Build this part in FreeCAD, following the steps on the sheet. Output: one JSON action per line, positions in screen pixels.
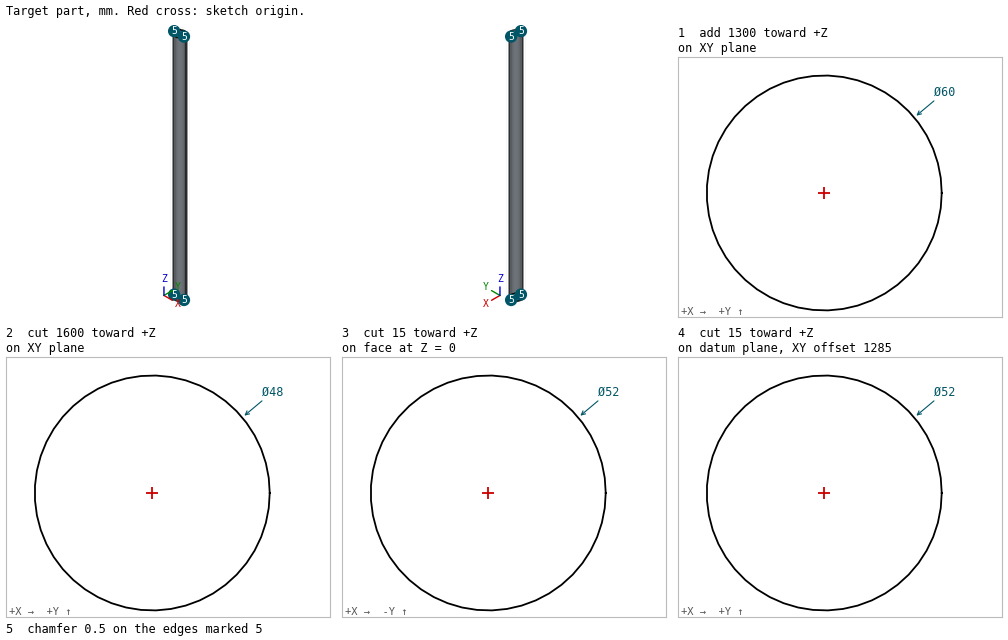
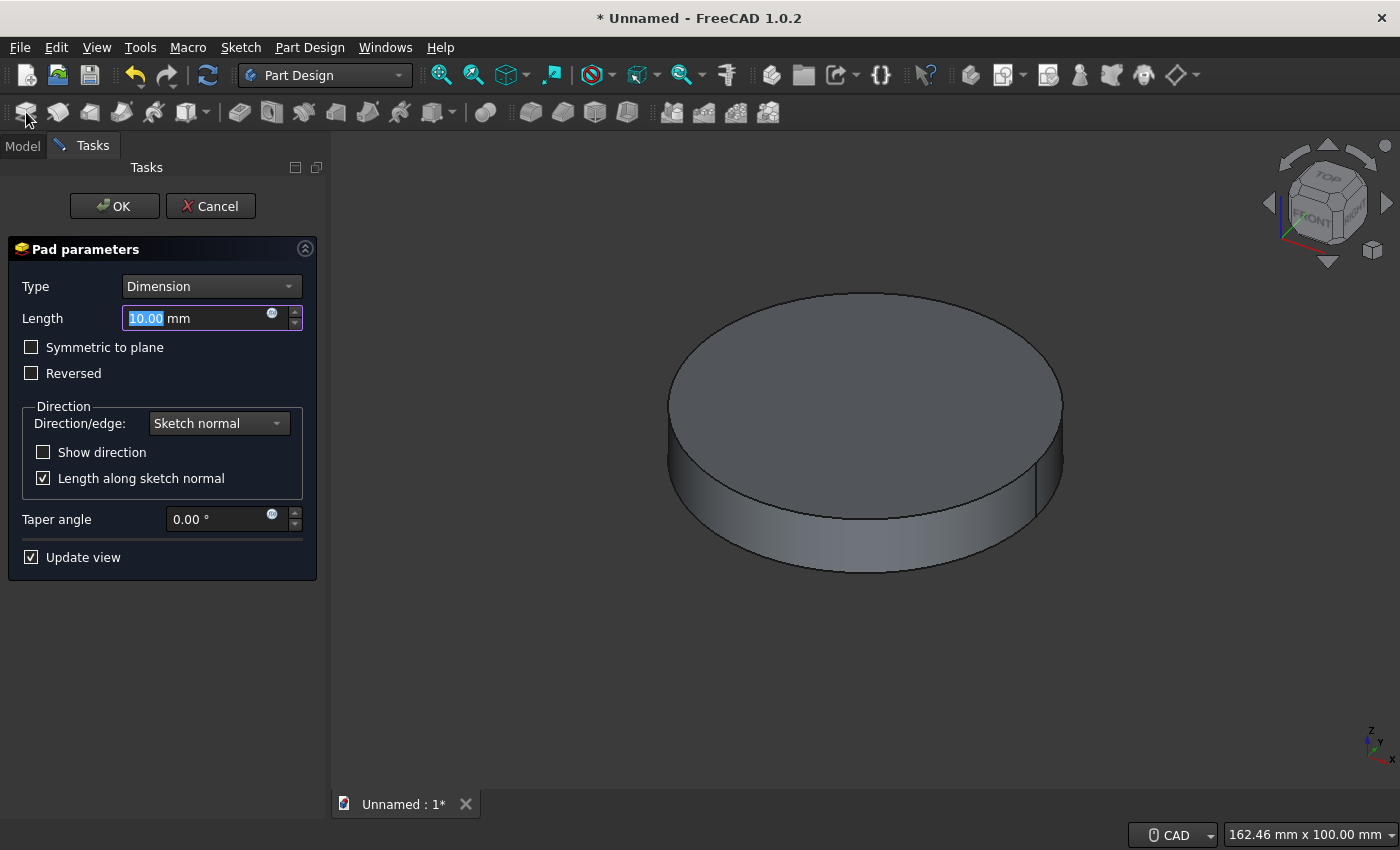
{"action": "type", "text": "1300"}
{"action": "key", "text": "Tab"}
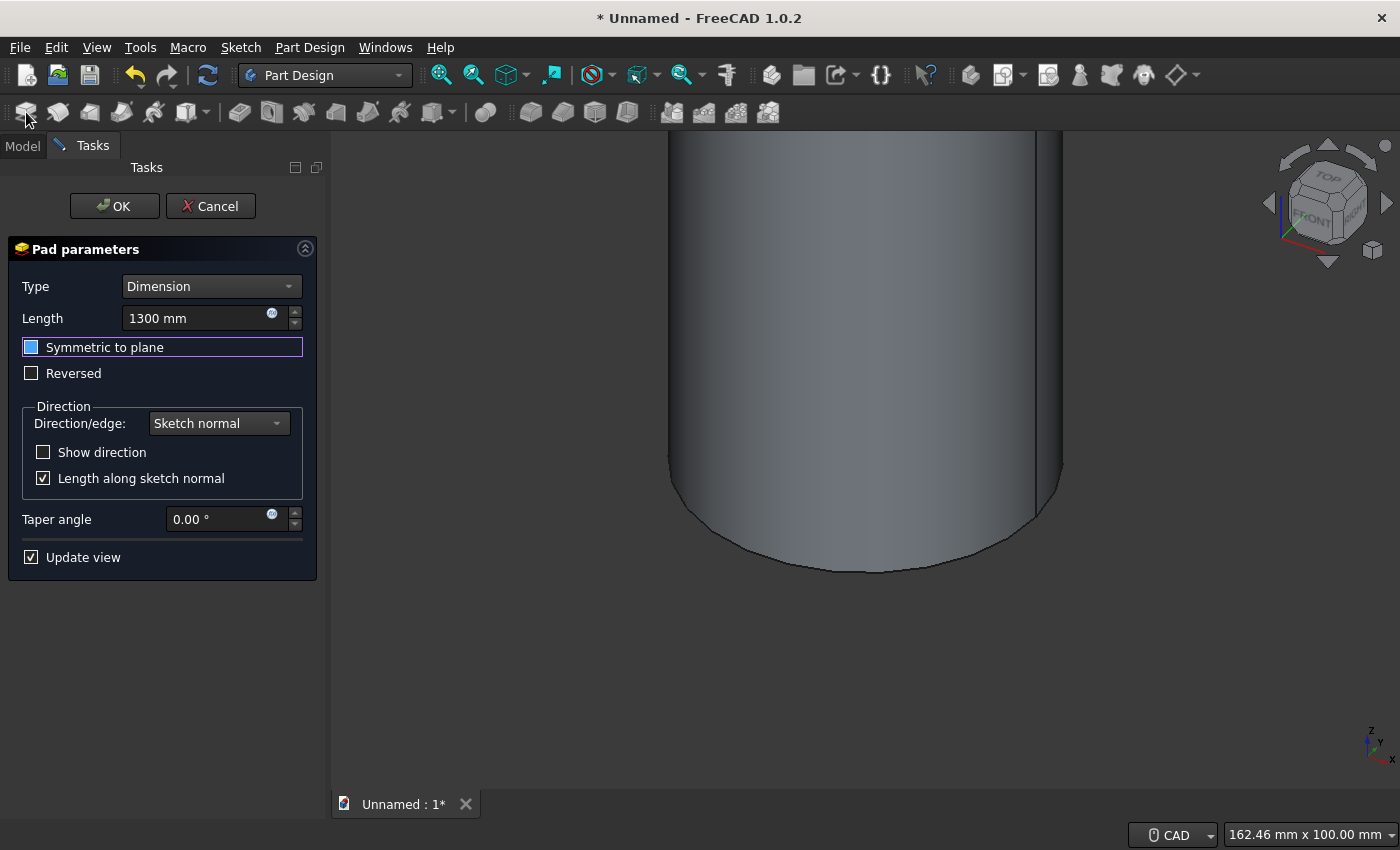
{"action": "left_click", "coordinate": [115, 206]}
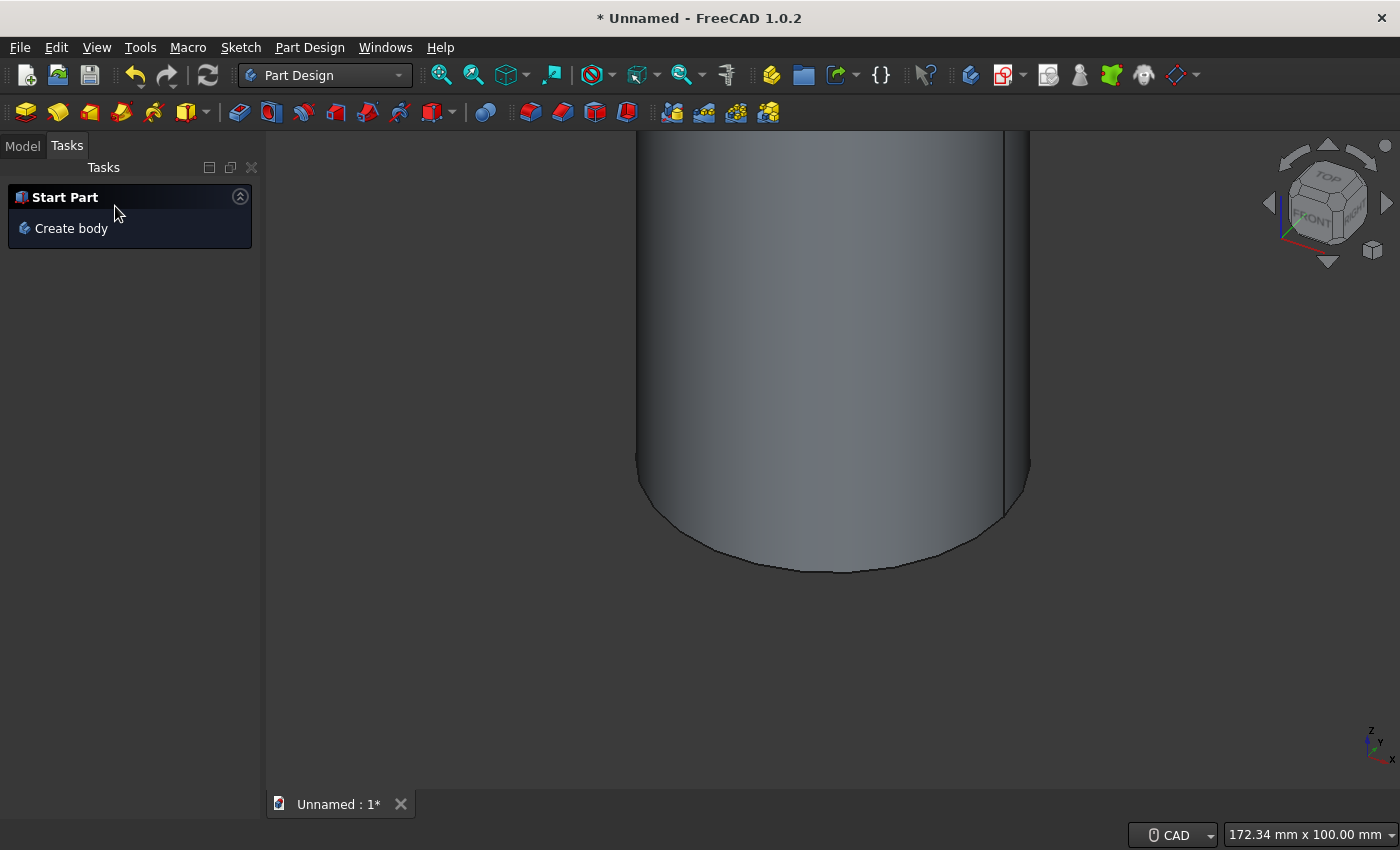
{"action": "left_click", "coordinate": [442, 76]}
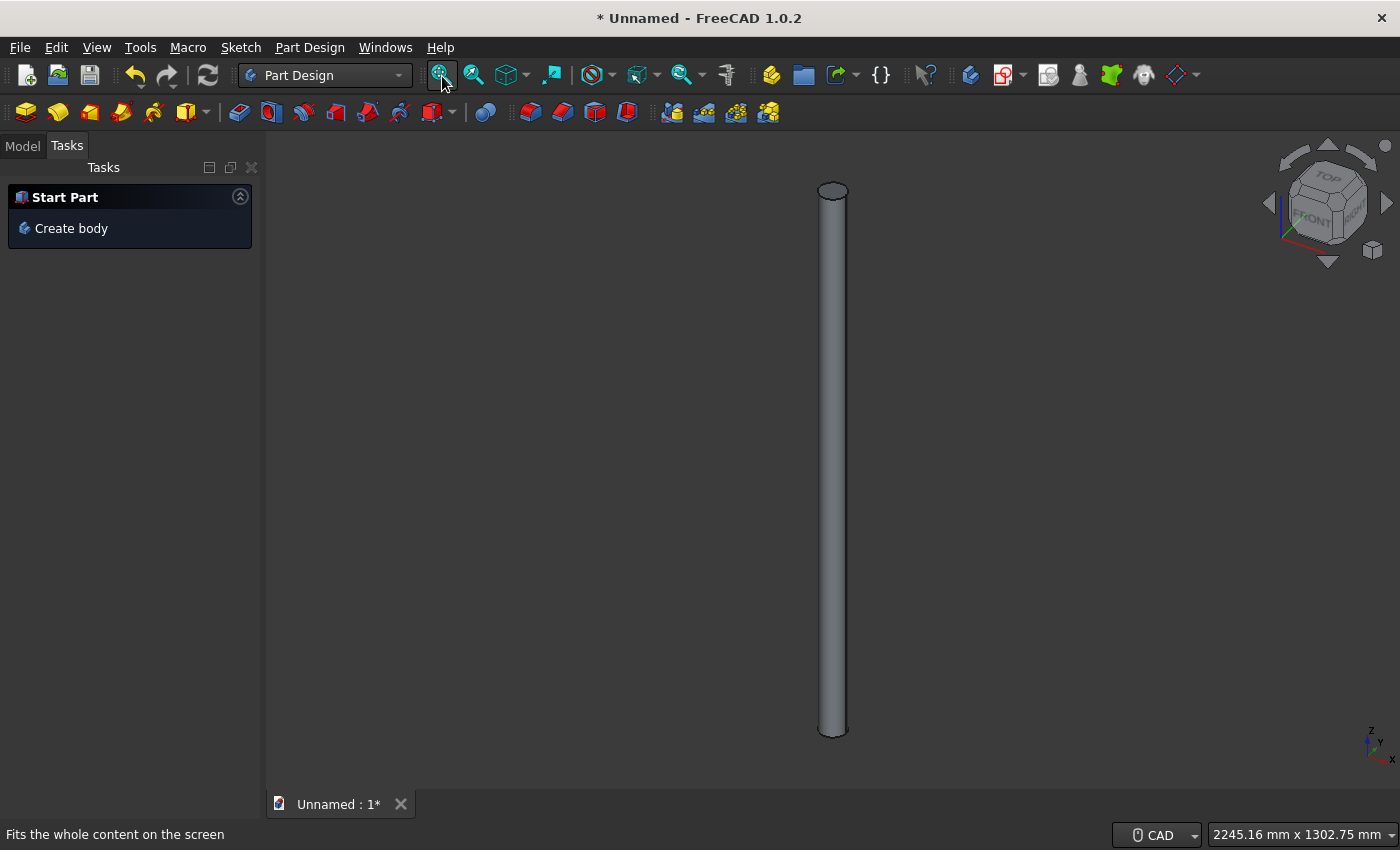
{"action": "left_click", "coordinate": [1004, 76]}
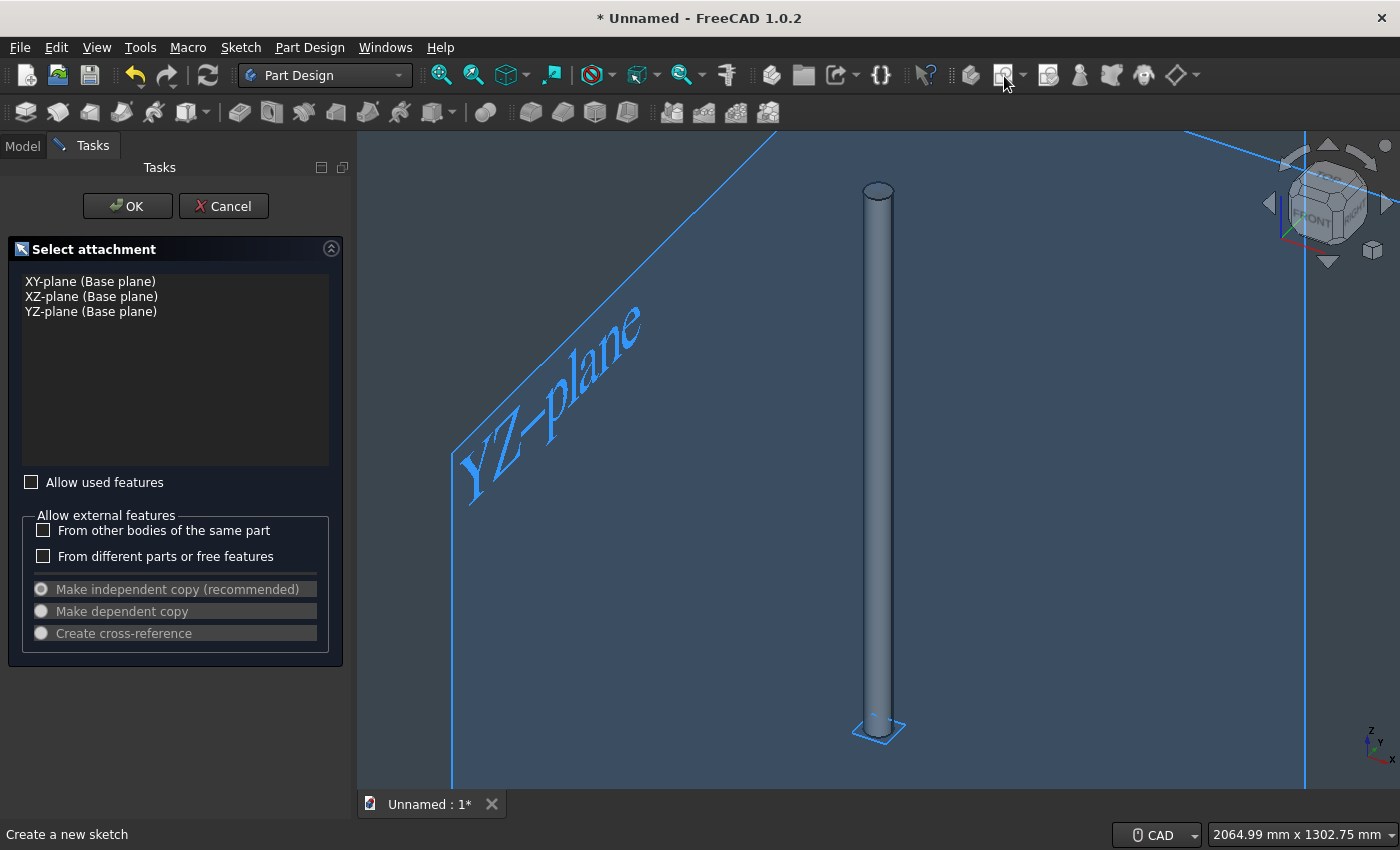
{"action": "left_click", "coordinate": [82, 282]}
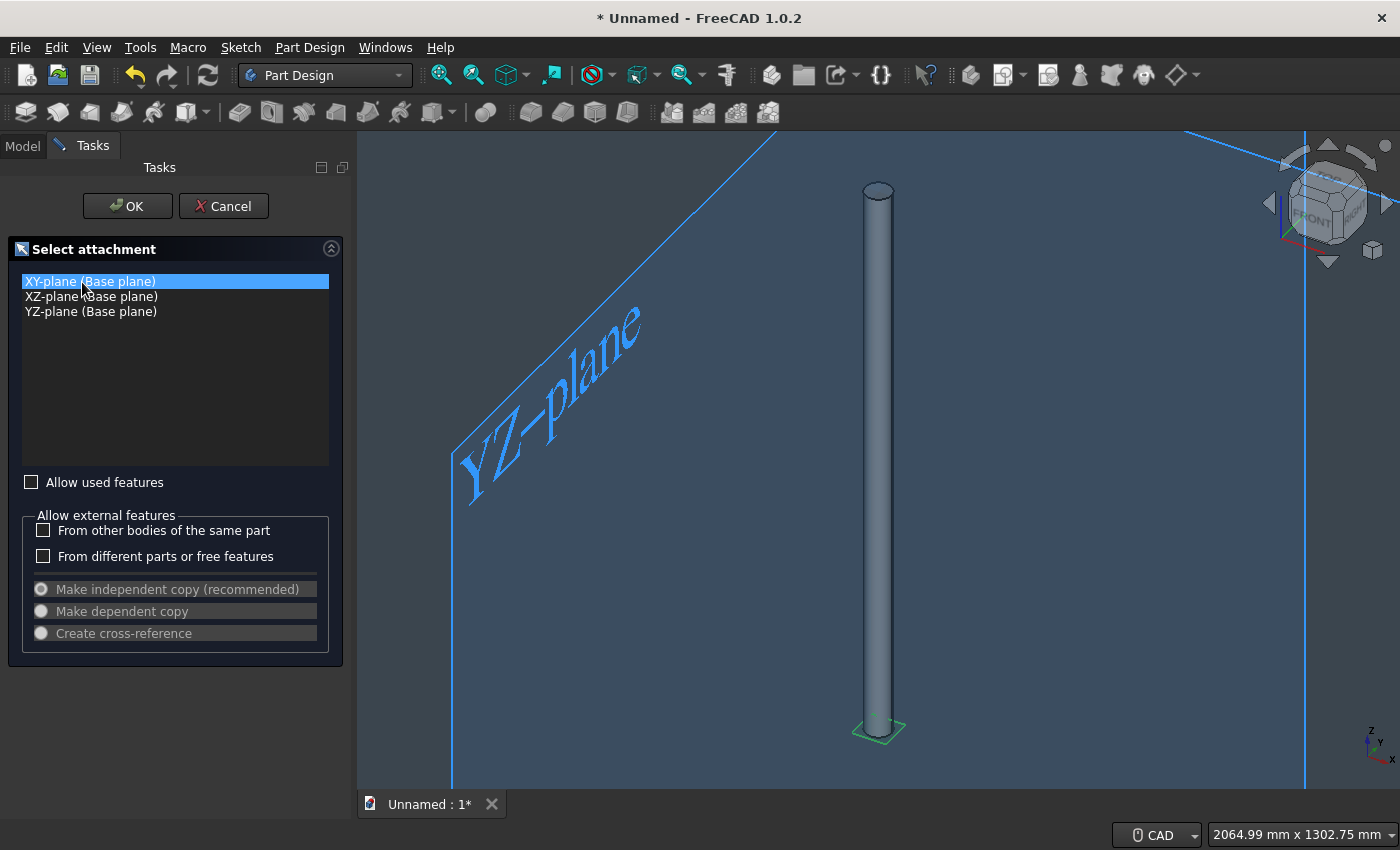
{"action": "left_click", "coordinate": [128, 206]}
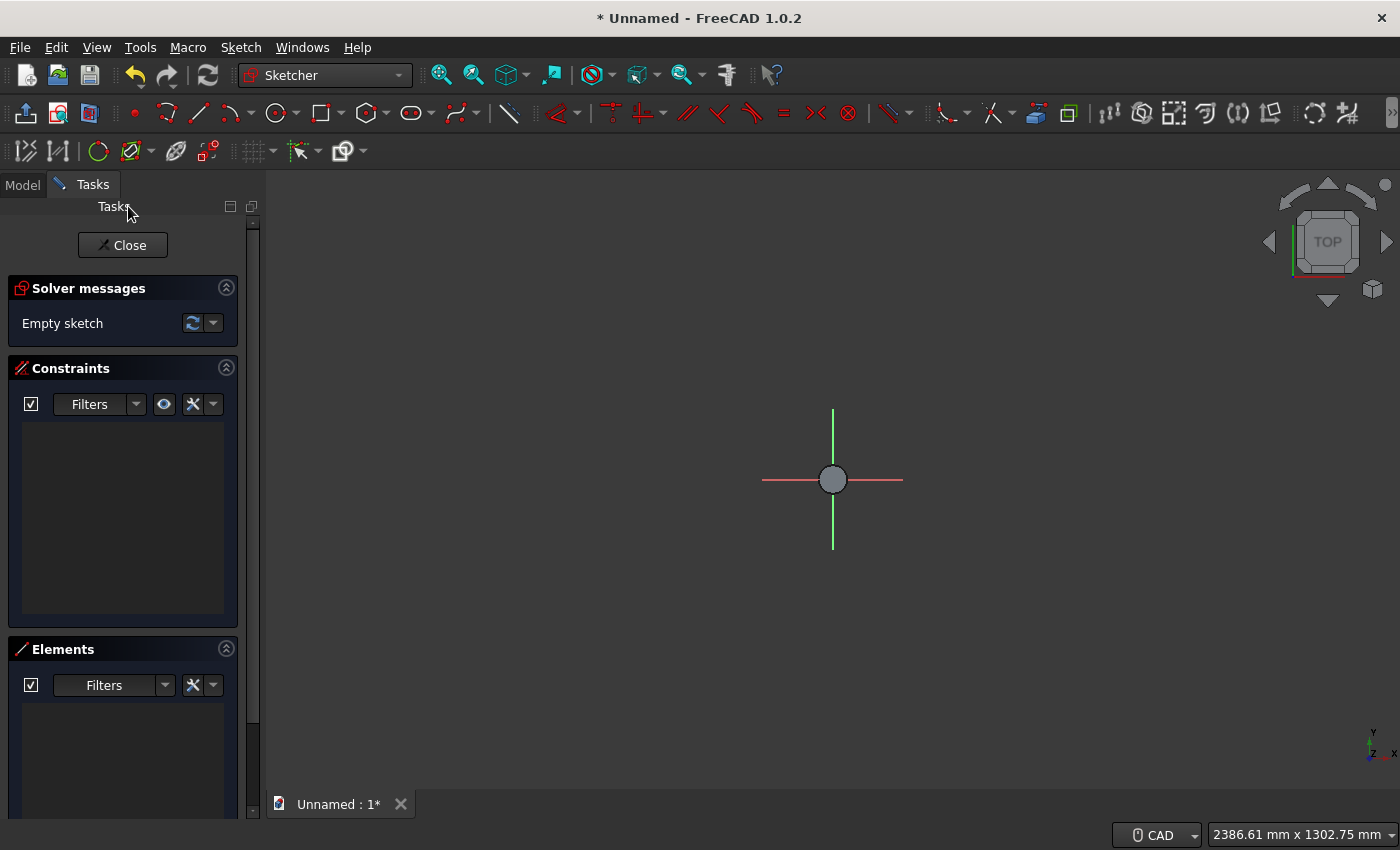
{"action": "left_click", "coordinate": [90, 114]}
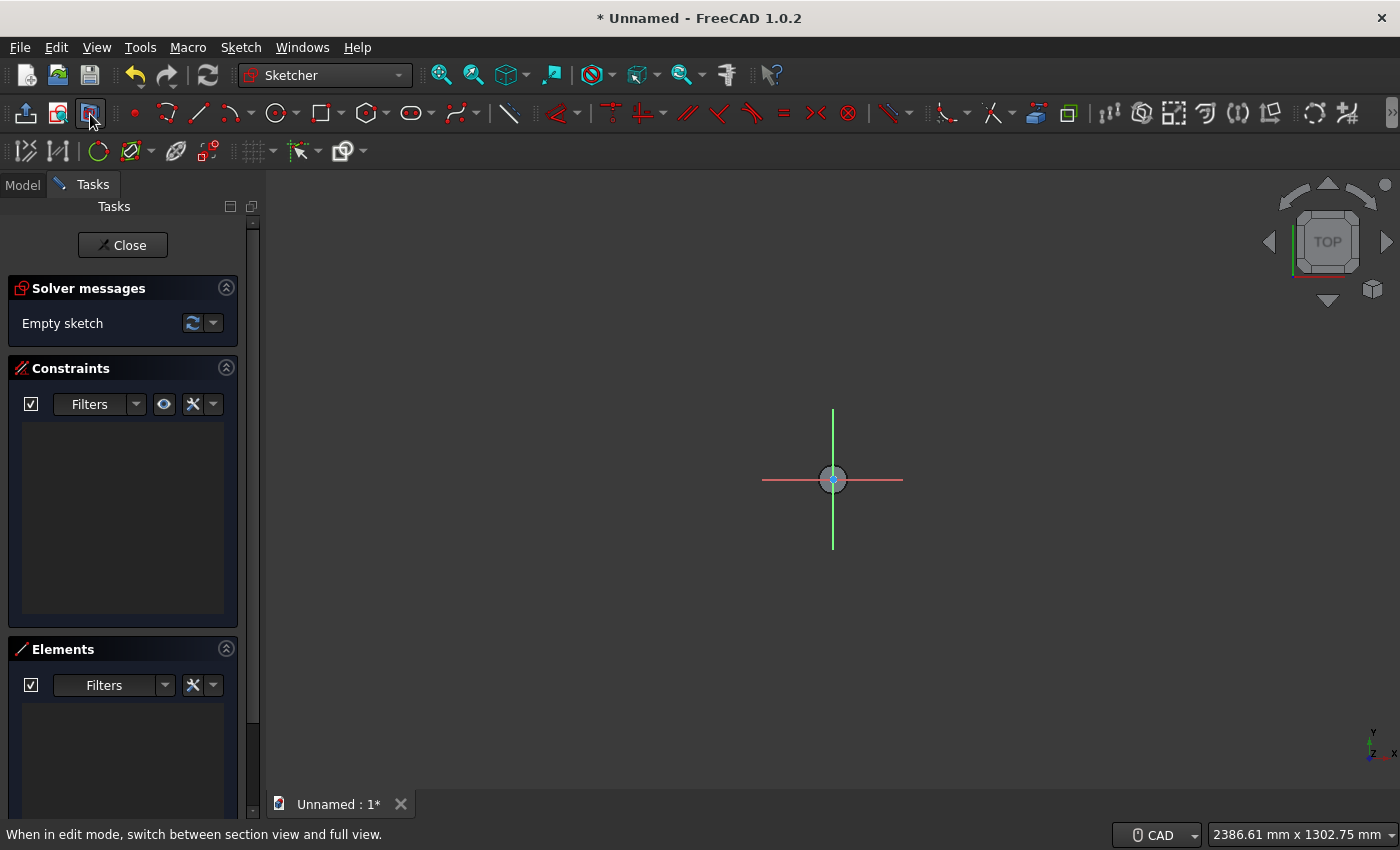
{"action": "scroll", "coordinate": [837, 480], "scroll_direction": "up", "scroll_amount": 14}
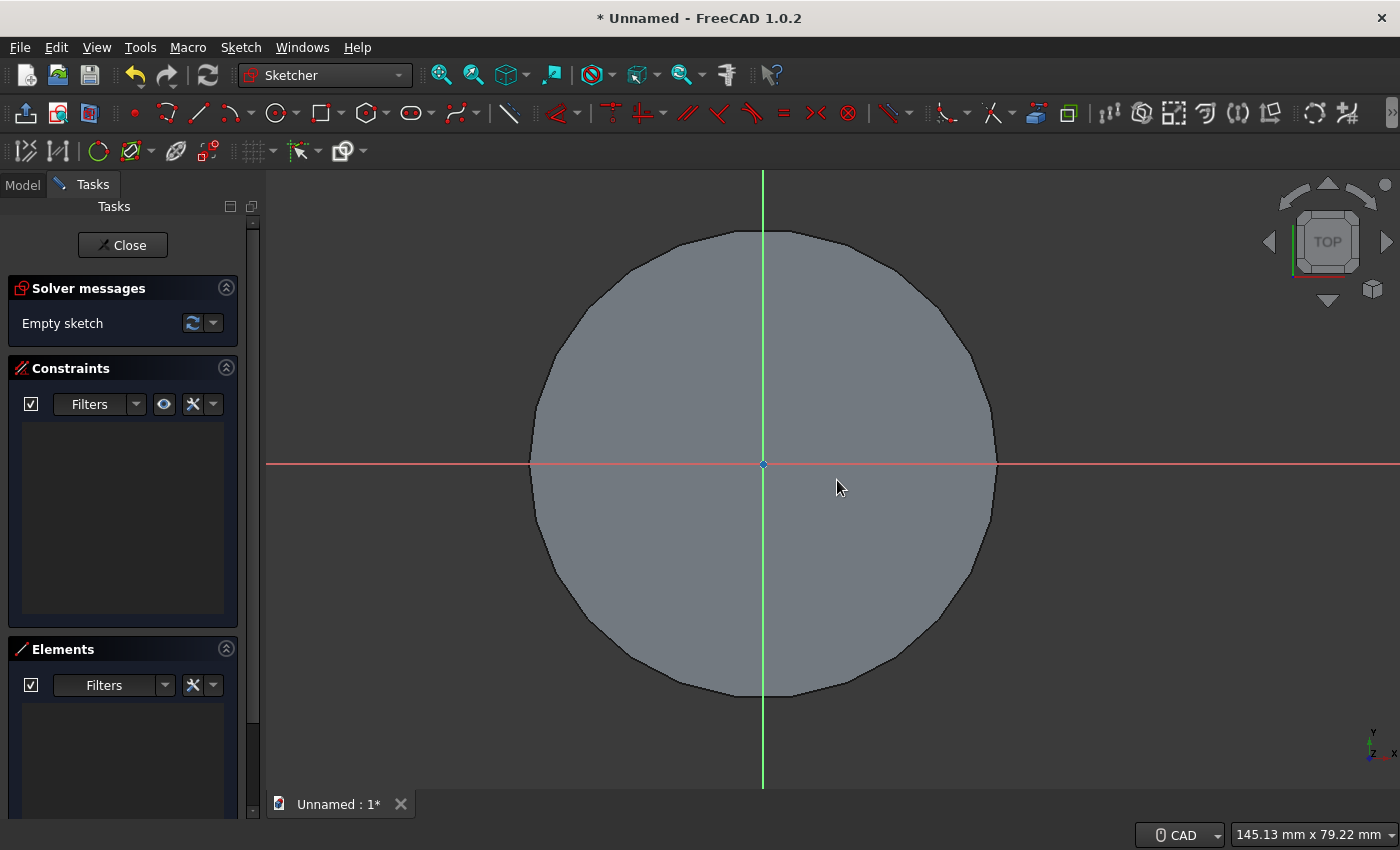
{"action": "left_click", "coordinate": [276, 114]}